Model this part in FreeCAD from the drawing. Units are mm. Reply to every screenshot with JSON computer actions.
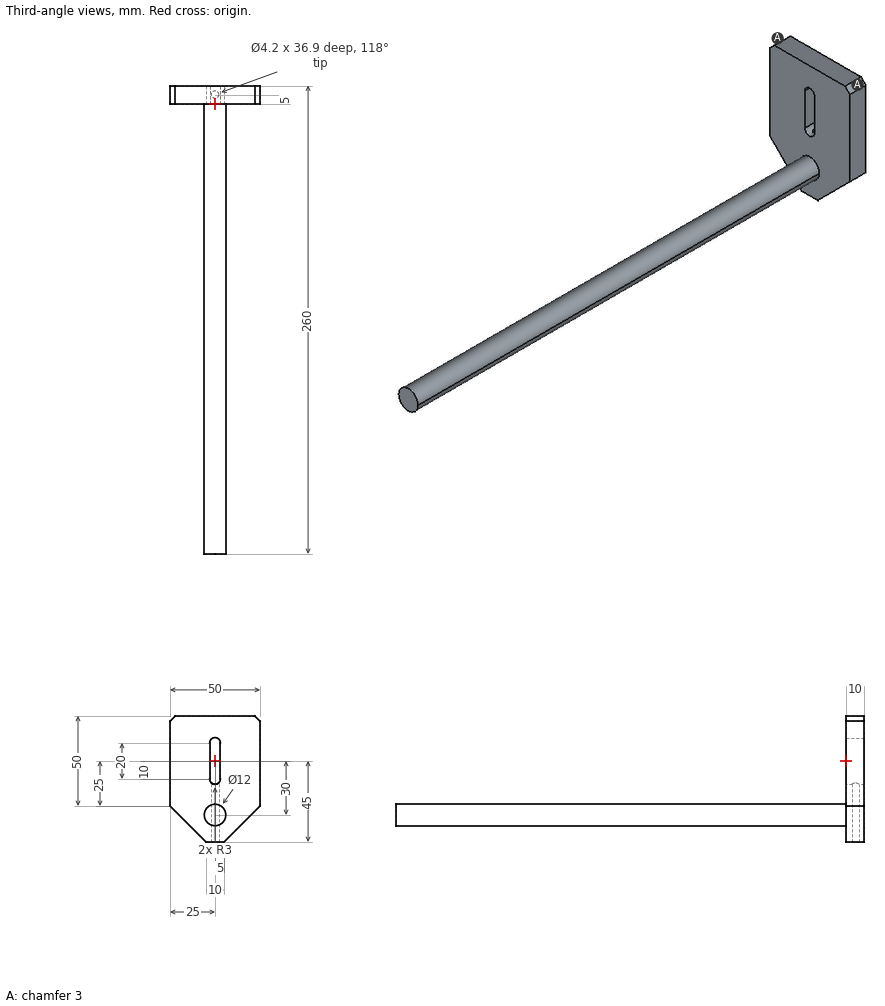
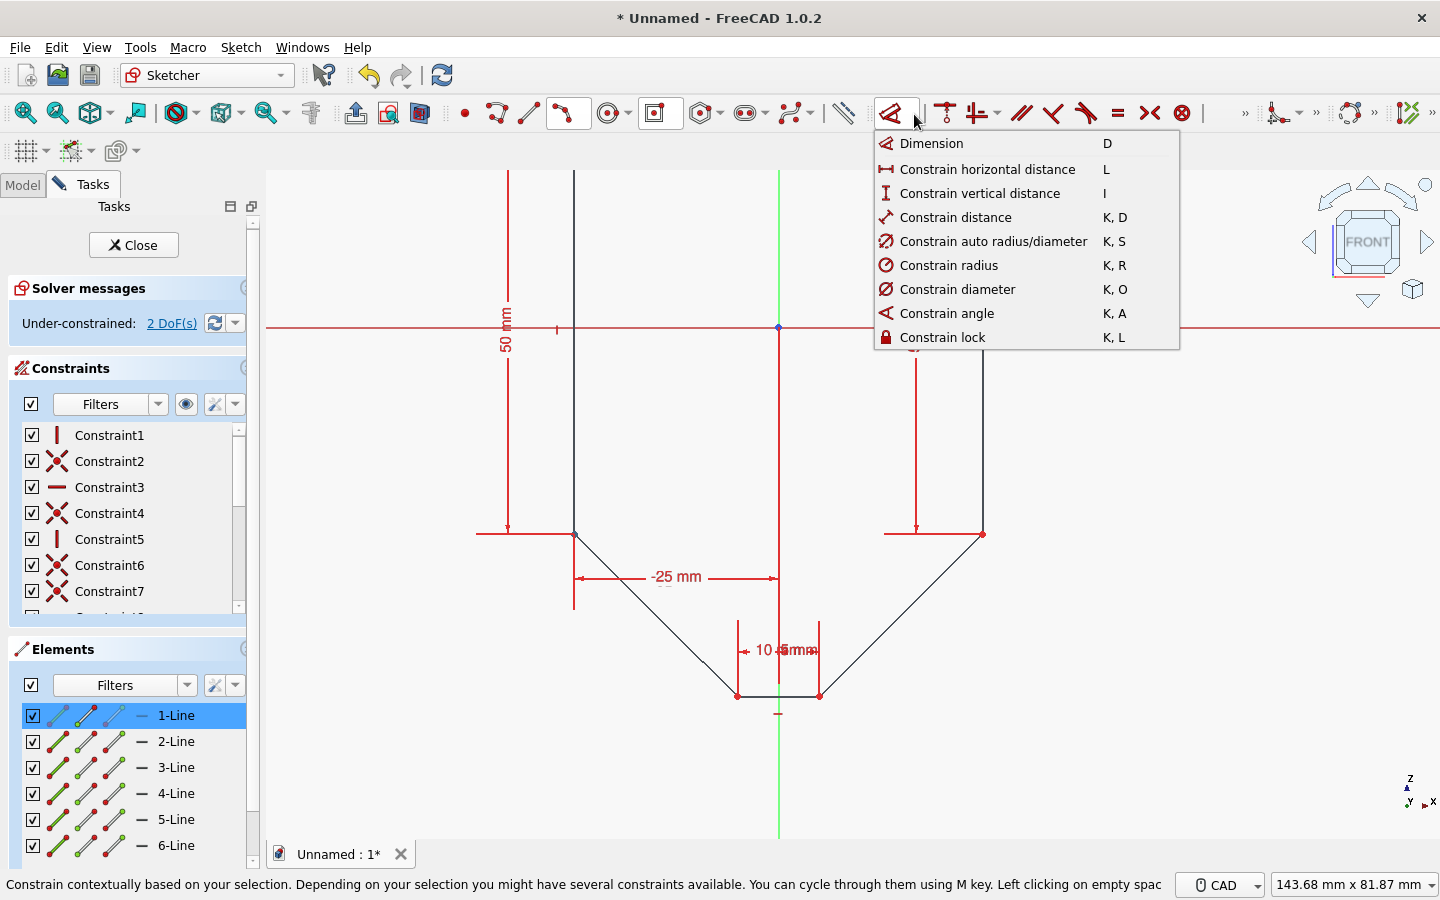
{"action": "left_click", "coordinate": [1027, 193]}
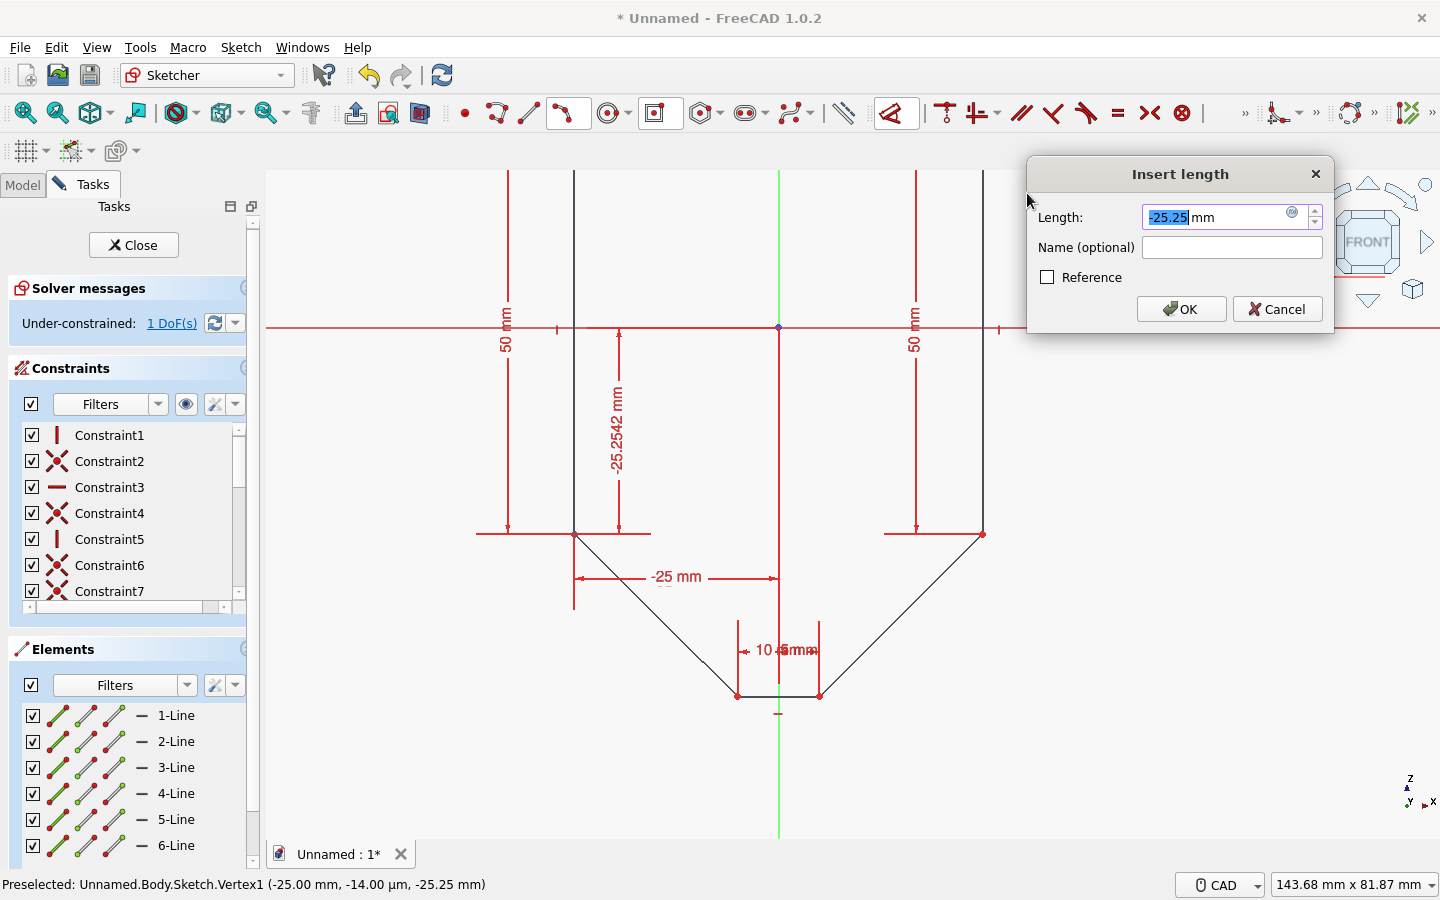
{"action": "type", "text": "-25"}
{"action": "key", "text": "Return"}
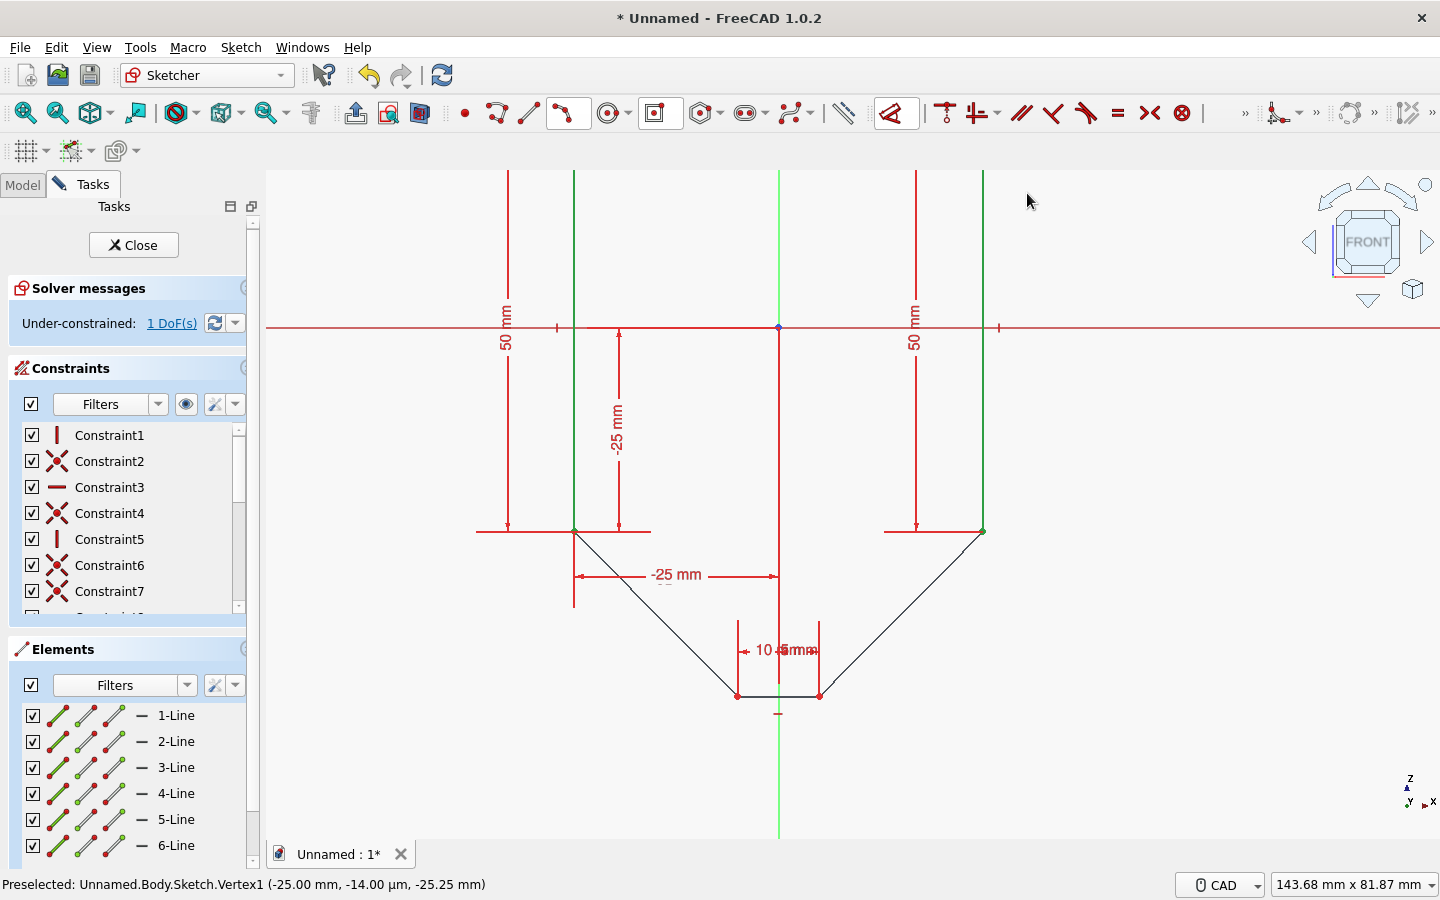
{"action": "left_click", "coordinate": [819, 697]}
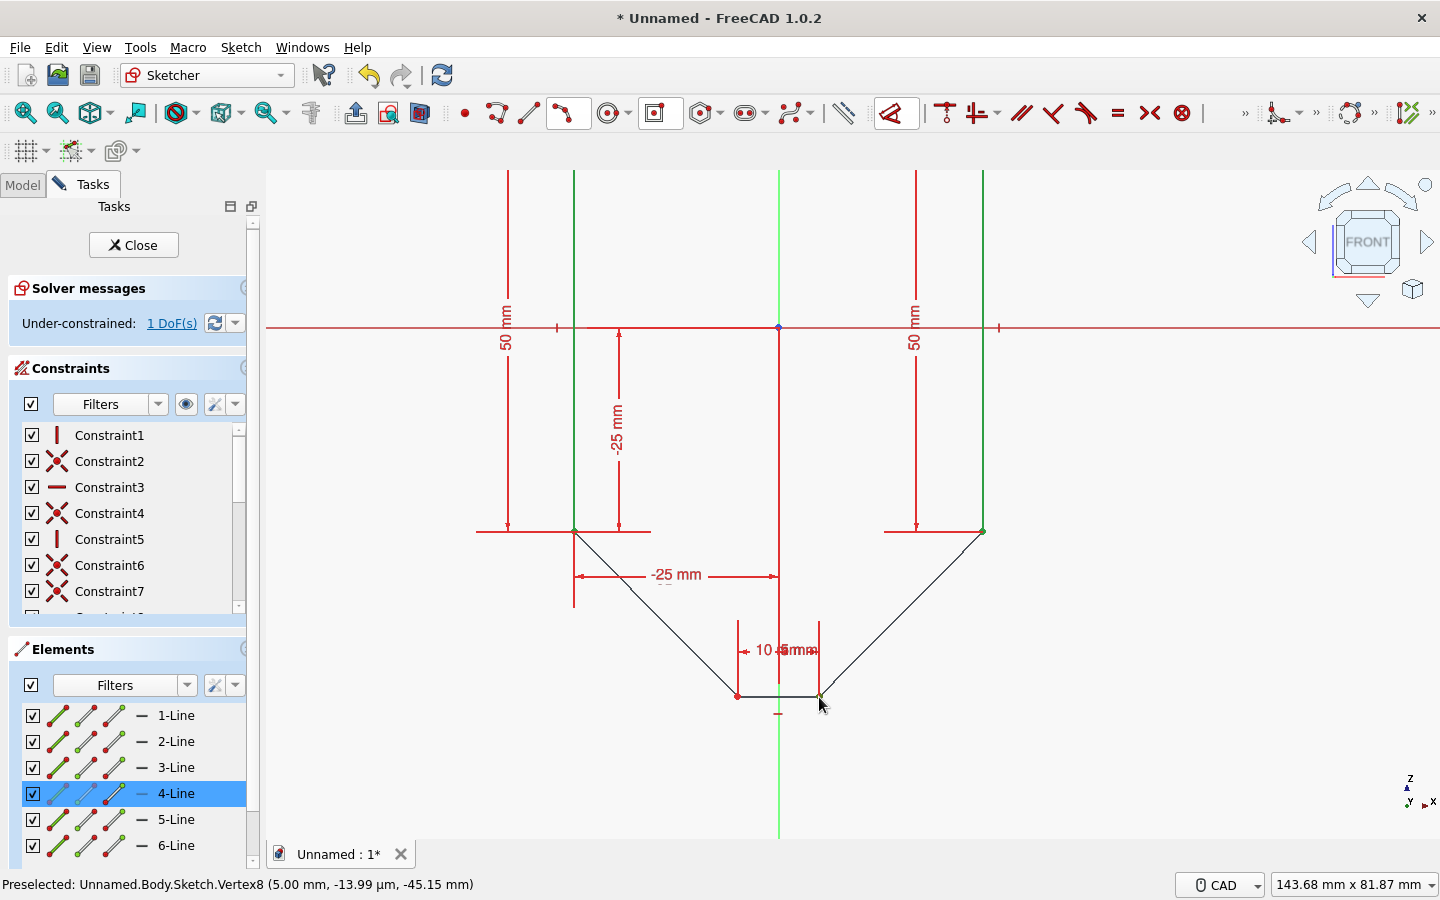
{"action": "key", "text": "i"}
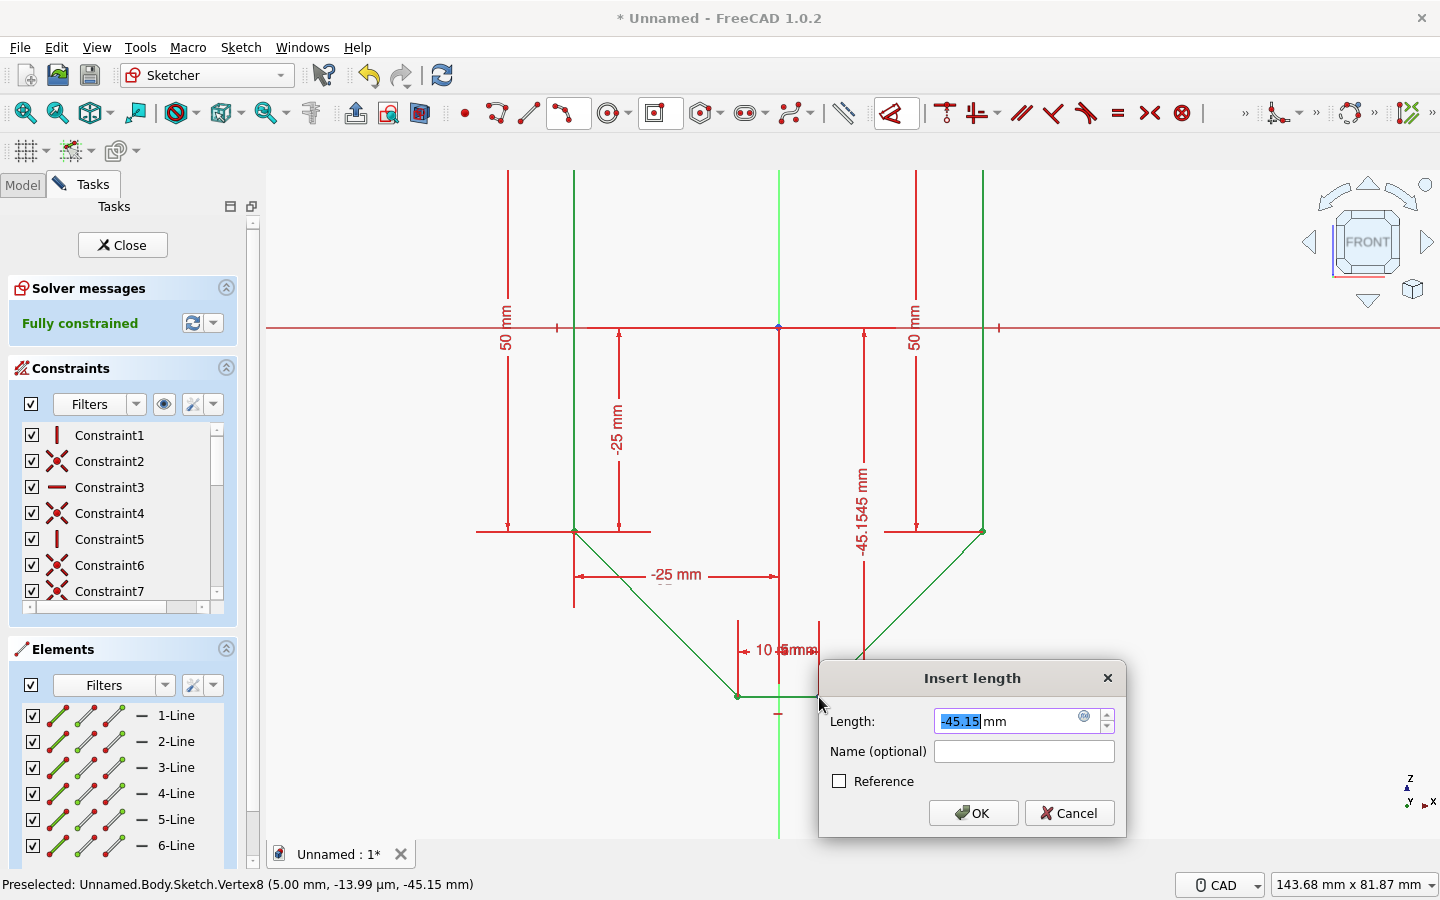
{"action": "type", "text": "-45"}
{"action": "key", "text": "Return"}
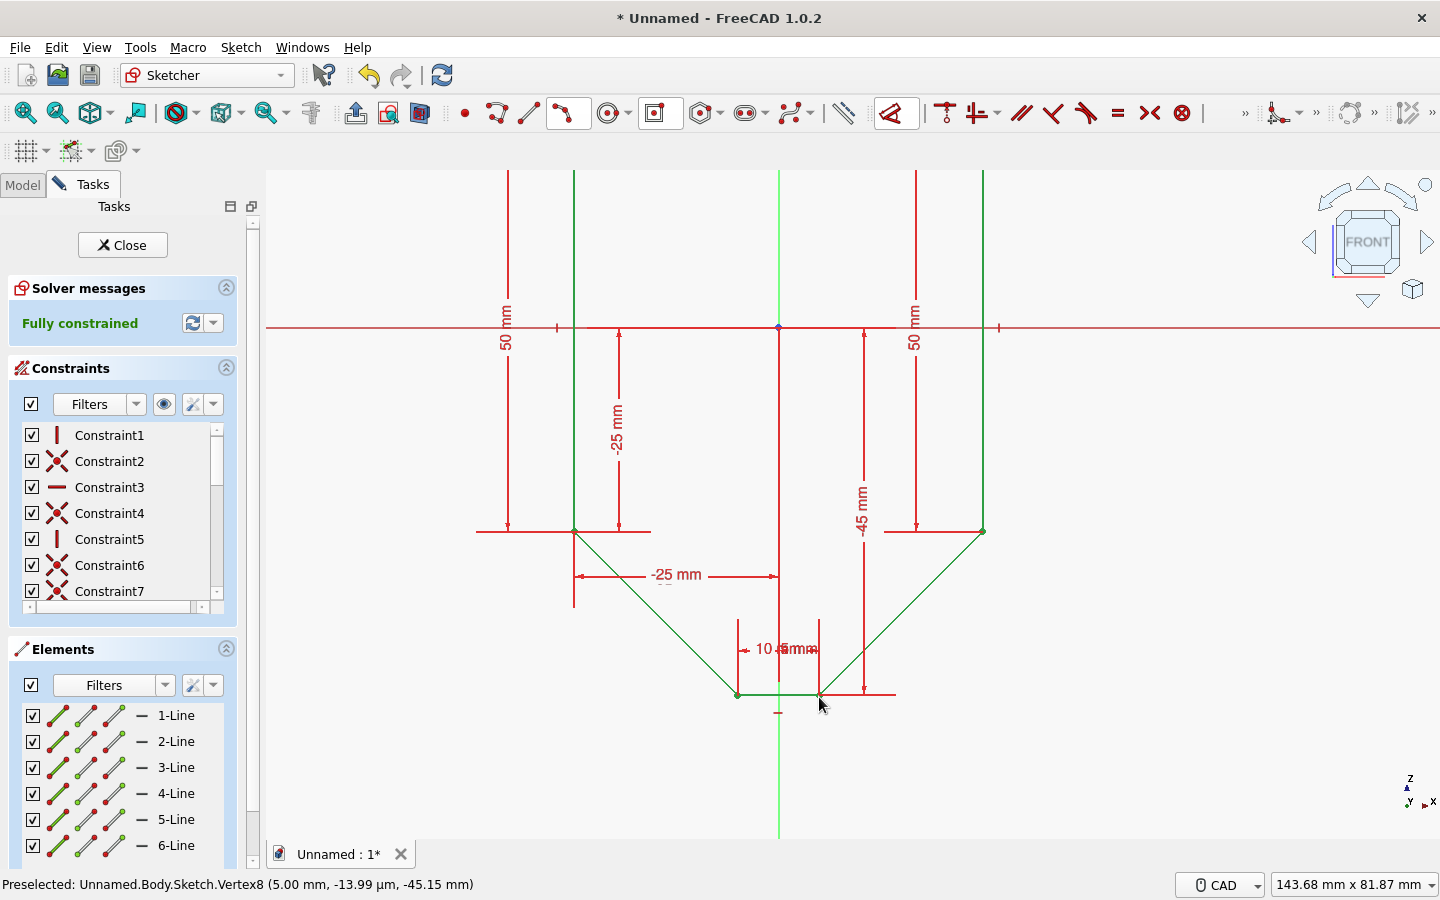
{"action": "left_click", "coordinate": [123, 245]}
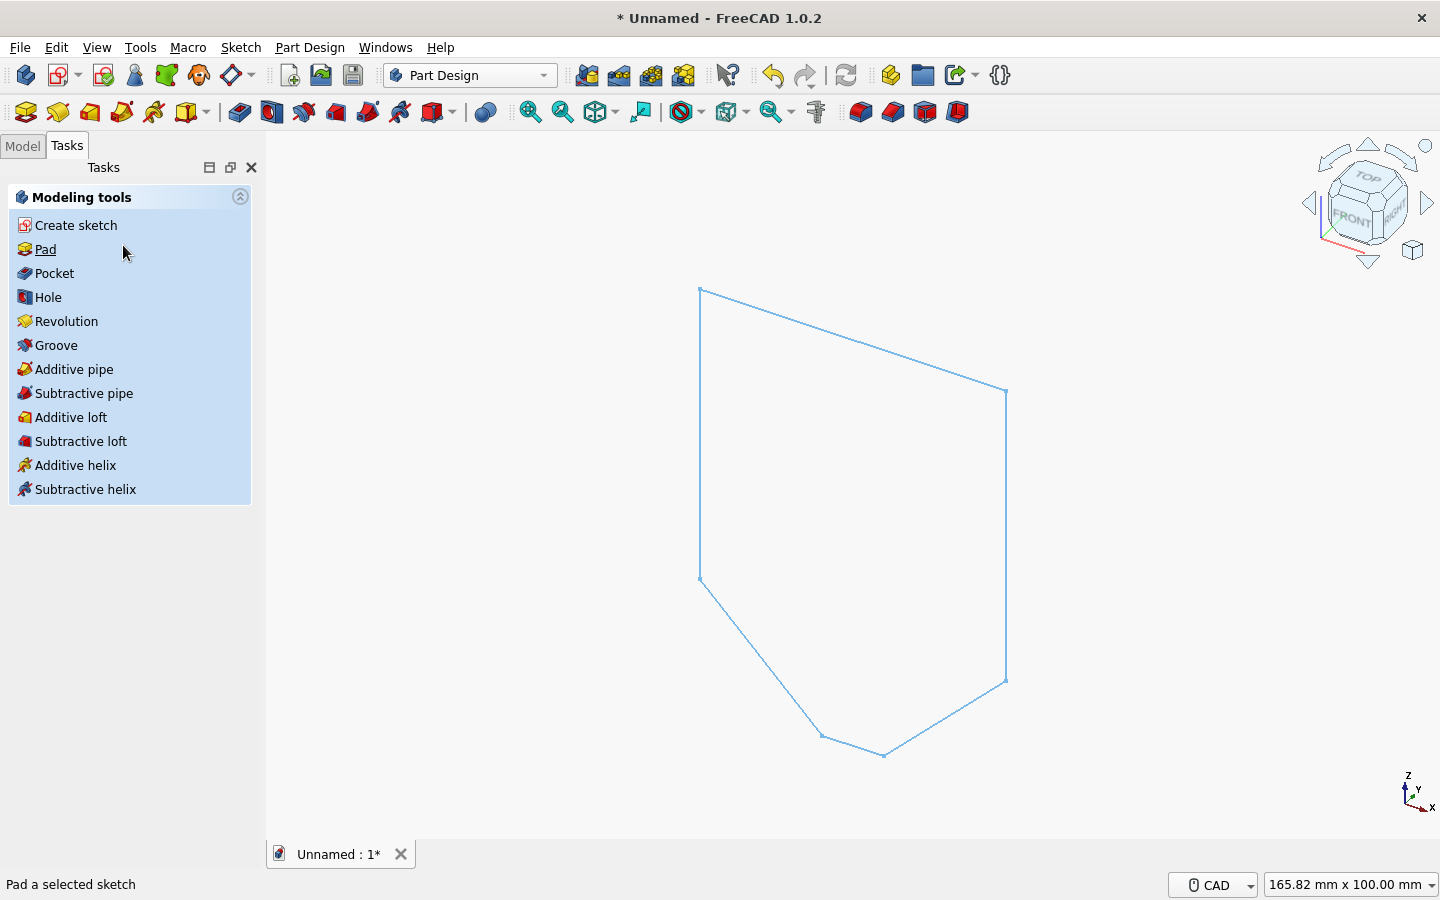
{"action": "left_click", "coordinate": [26, 112]}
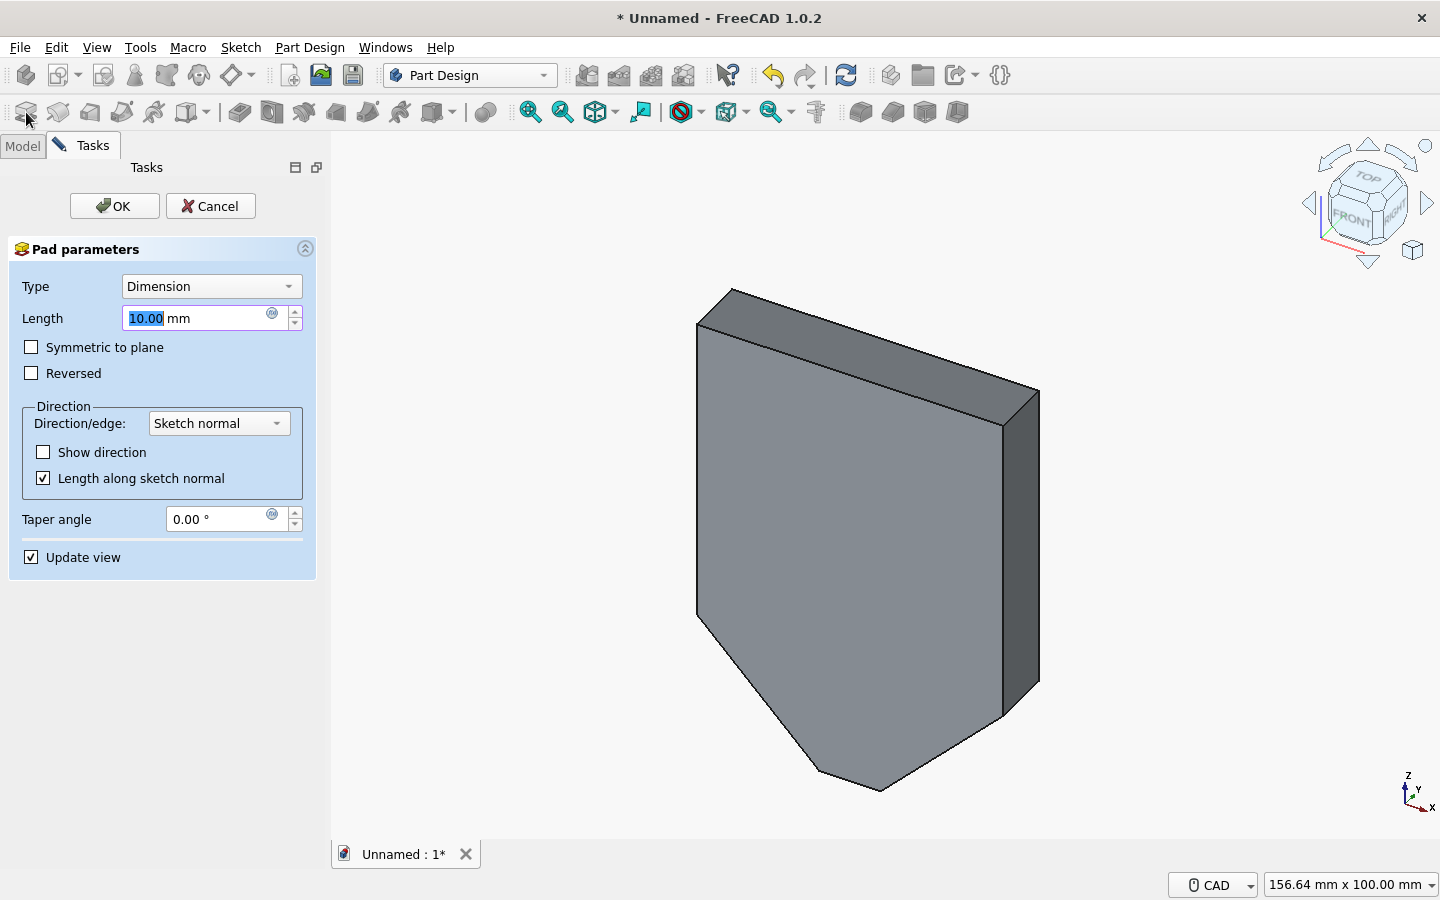
{"action": "type", "text": "10"}
{"action": "key", "text": "Tab"}